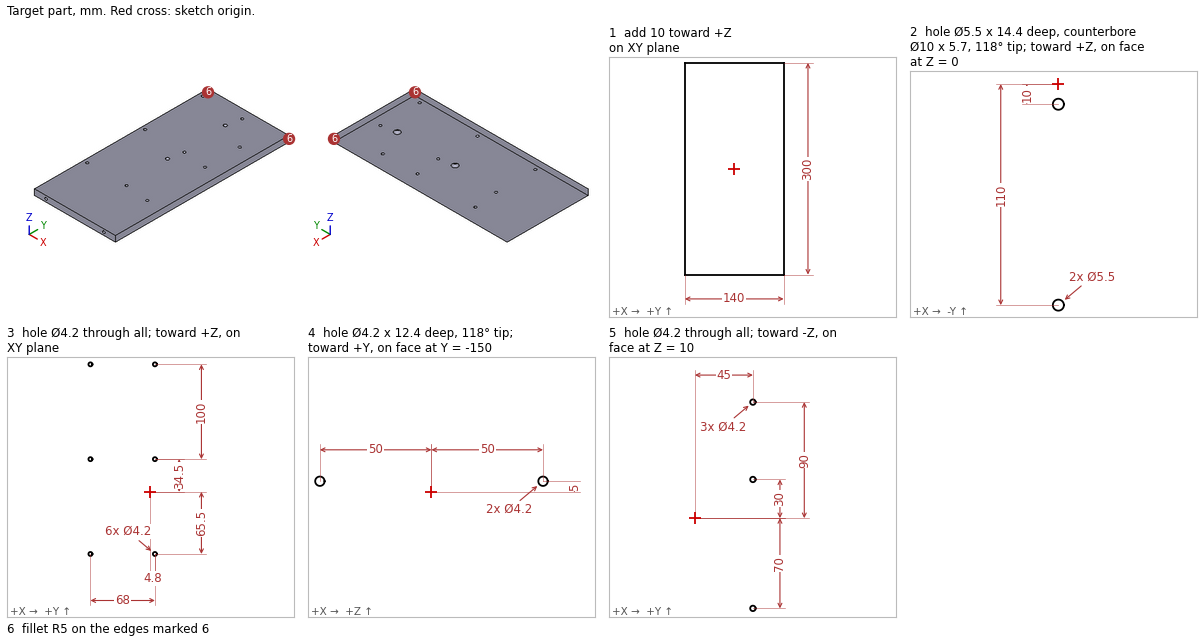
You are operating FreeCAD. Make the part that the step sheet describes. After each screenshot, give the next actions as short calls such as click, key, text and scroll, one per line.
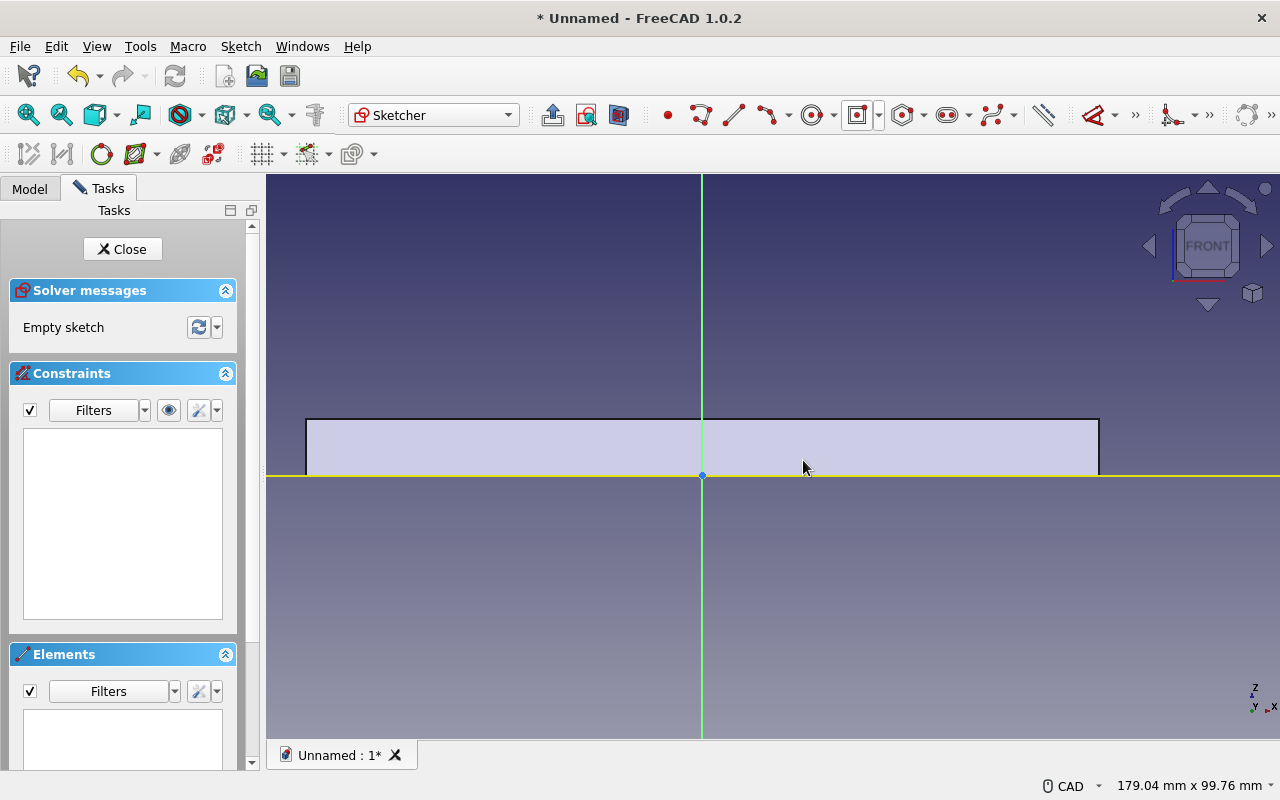
click(812, 116)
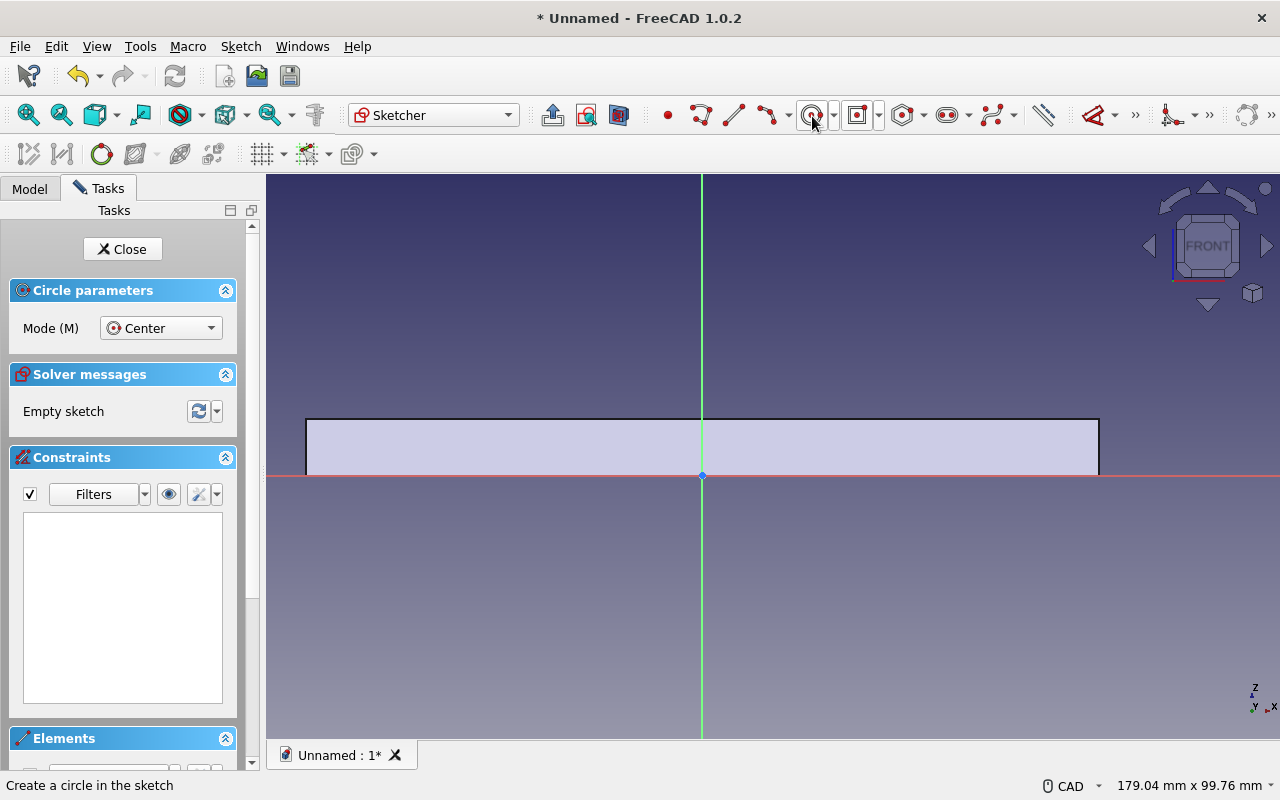
scroll(985, 447, up, 4)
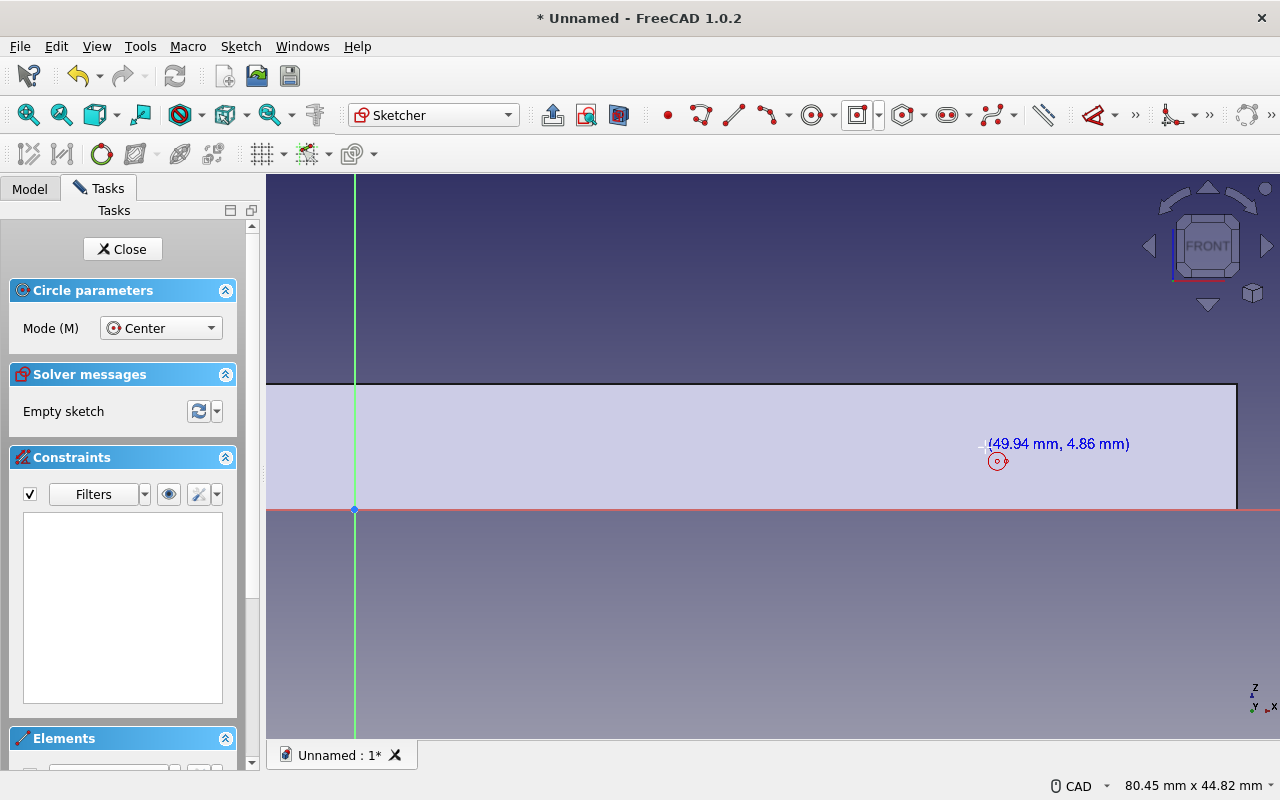
click(985, 447)
click(1004, 428)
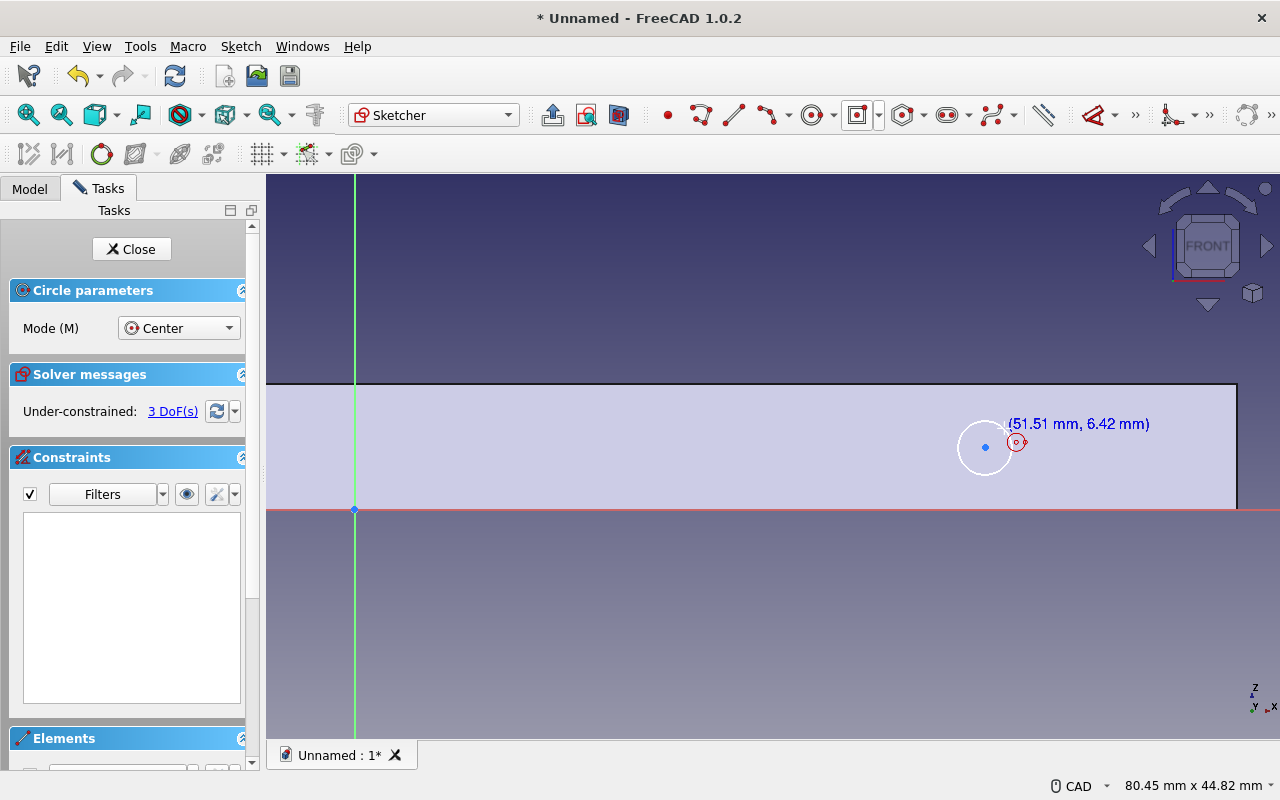
scroll(990, 449, down, 4)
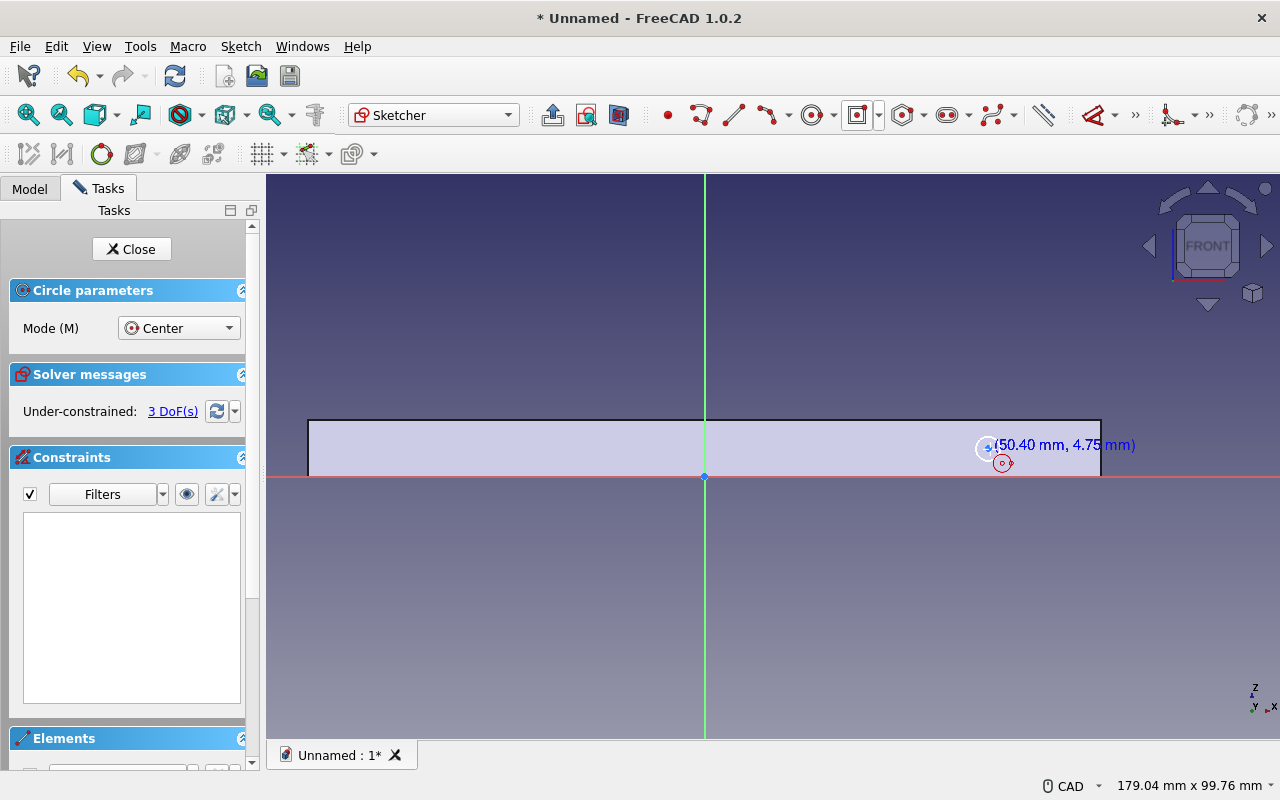
scroll(422, 448, up, 4)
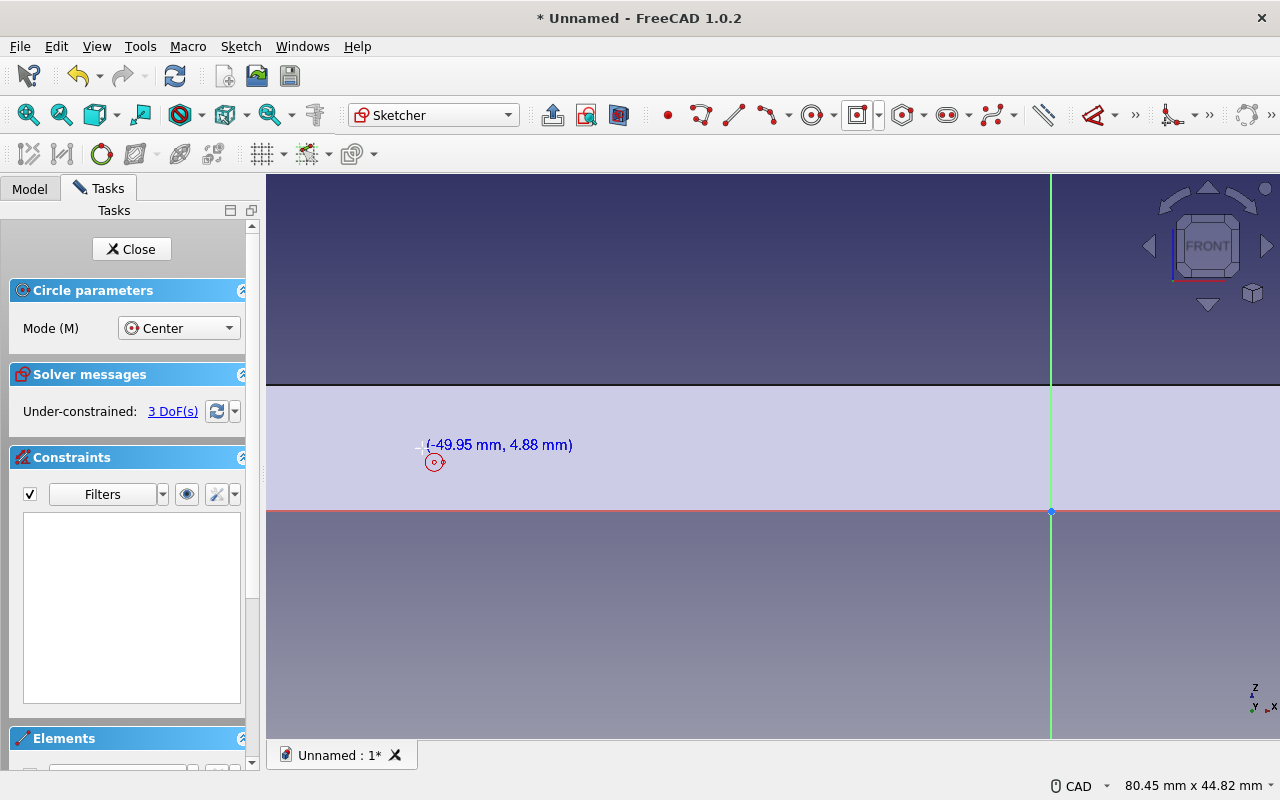
click(421, 448)
click(440, 429)
key(Escape)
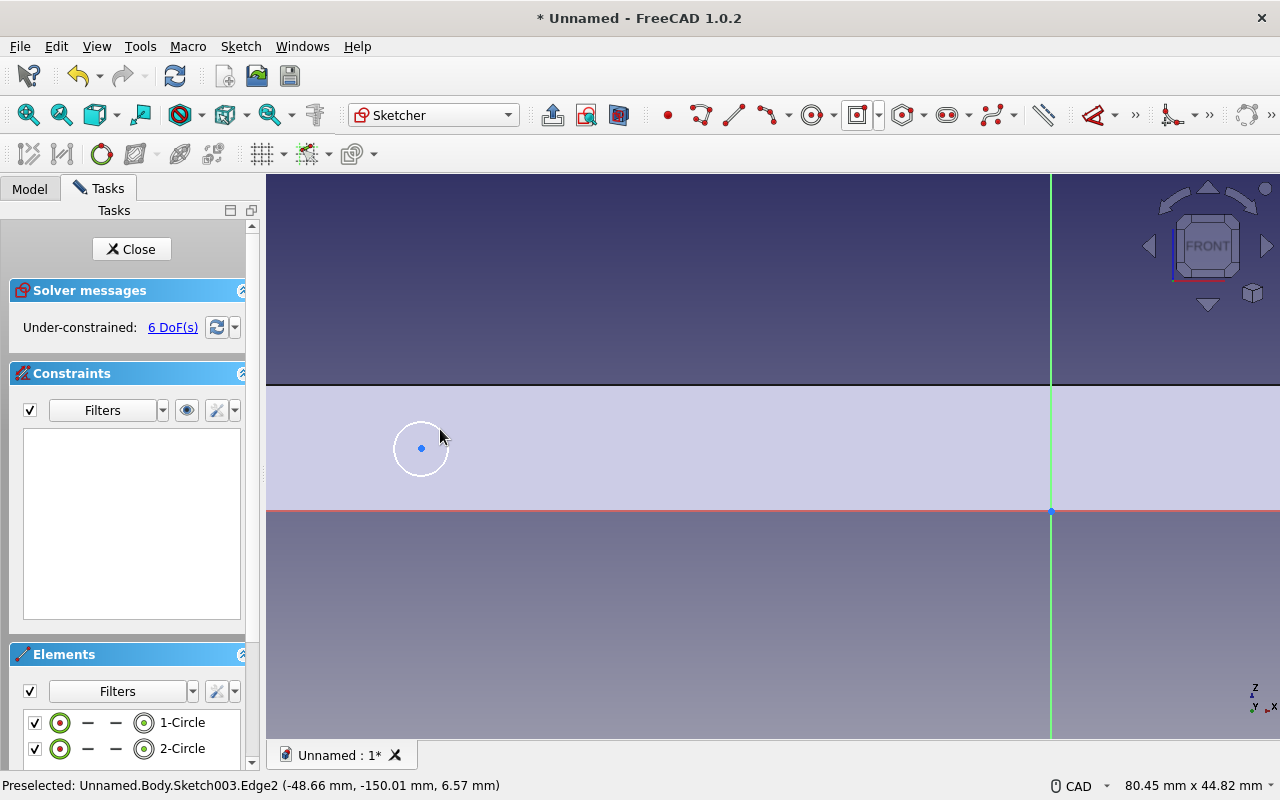
scroll(421, 448, down, 4)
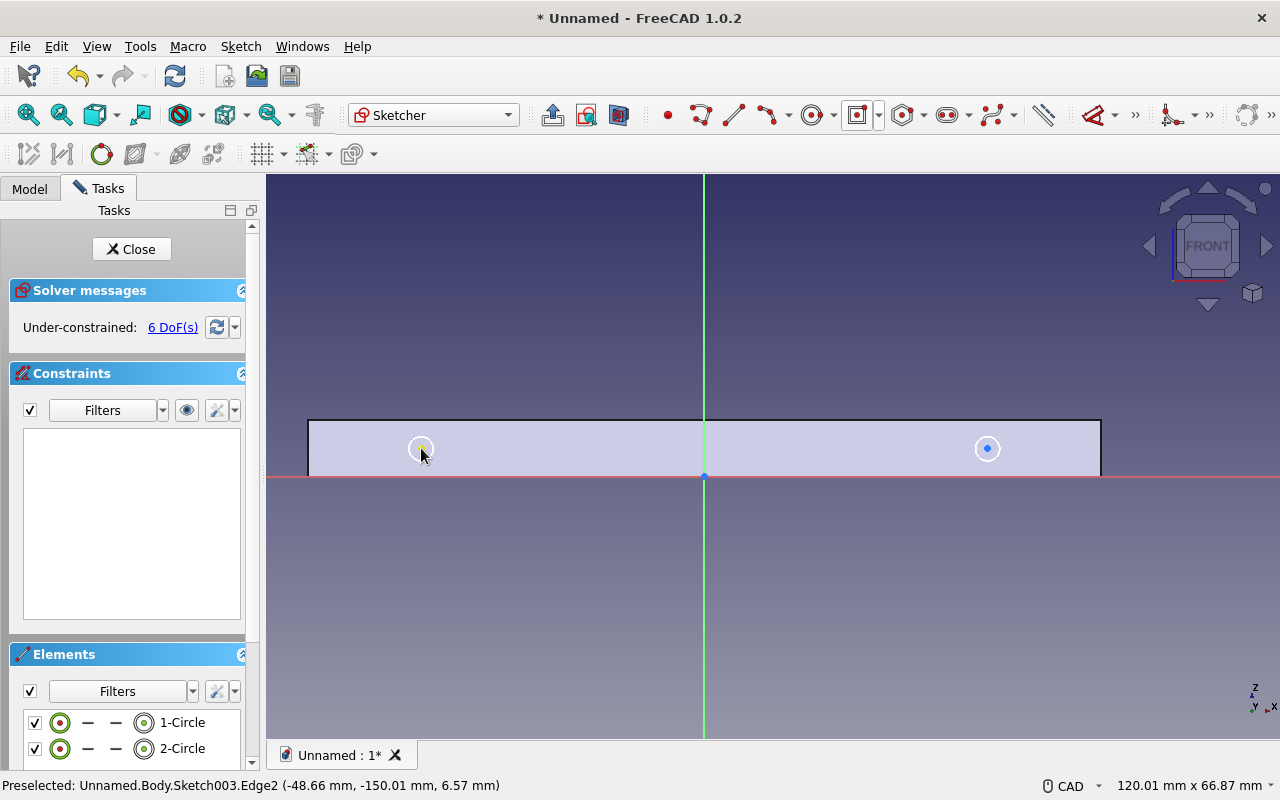
click(996, 440)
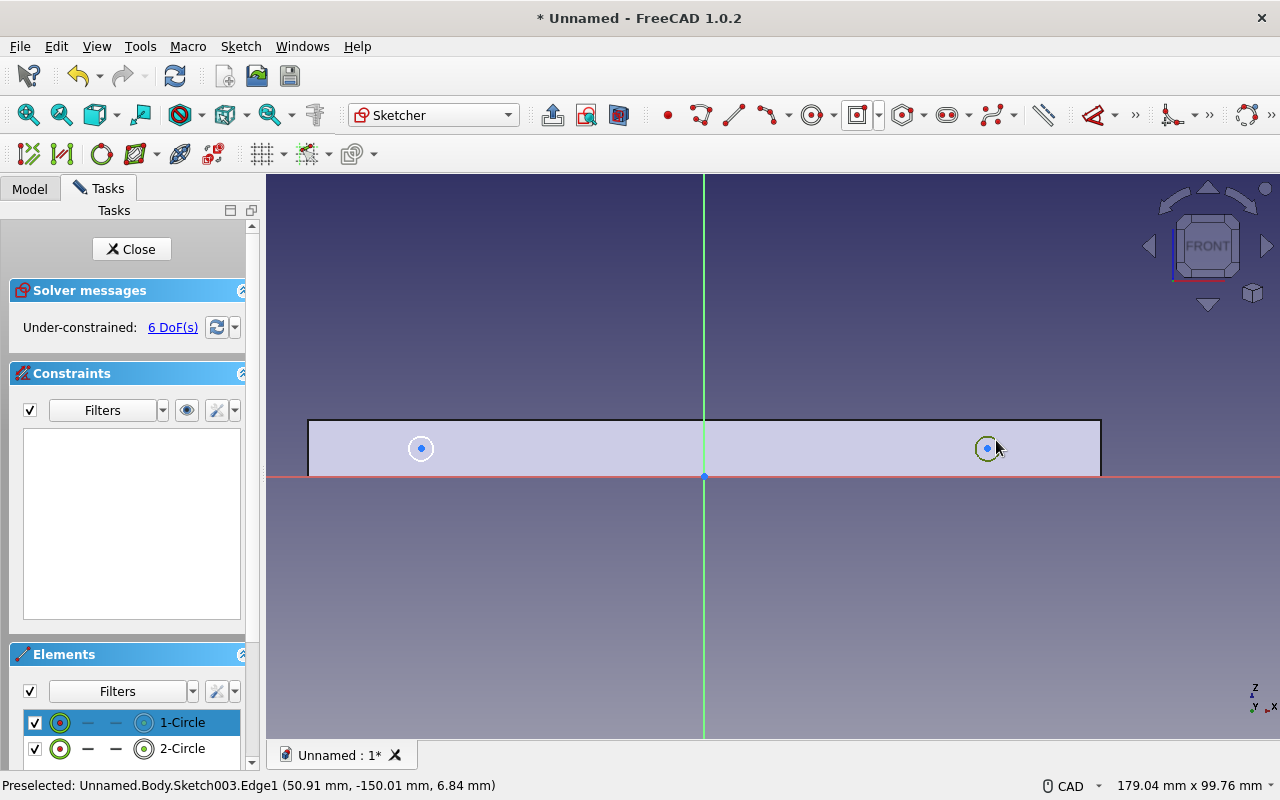
click(430, 440)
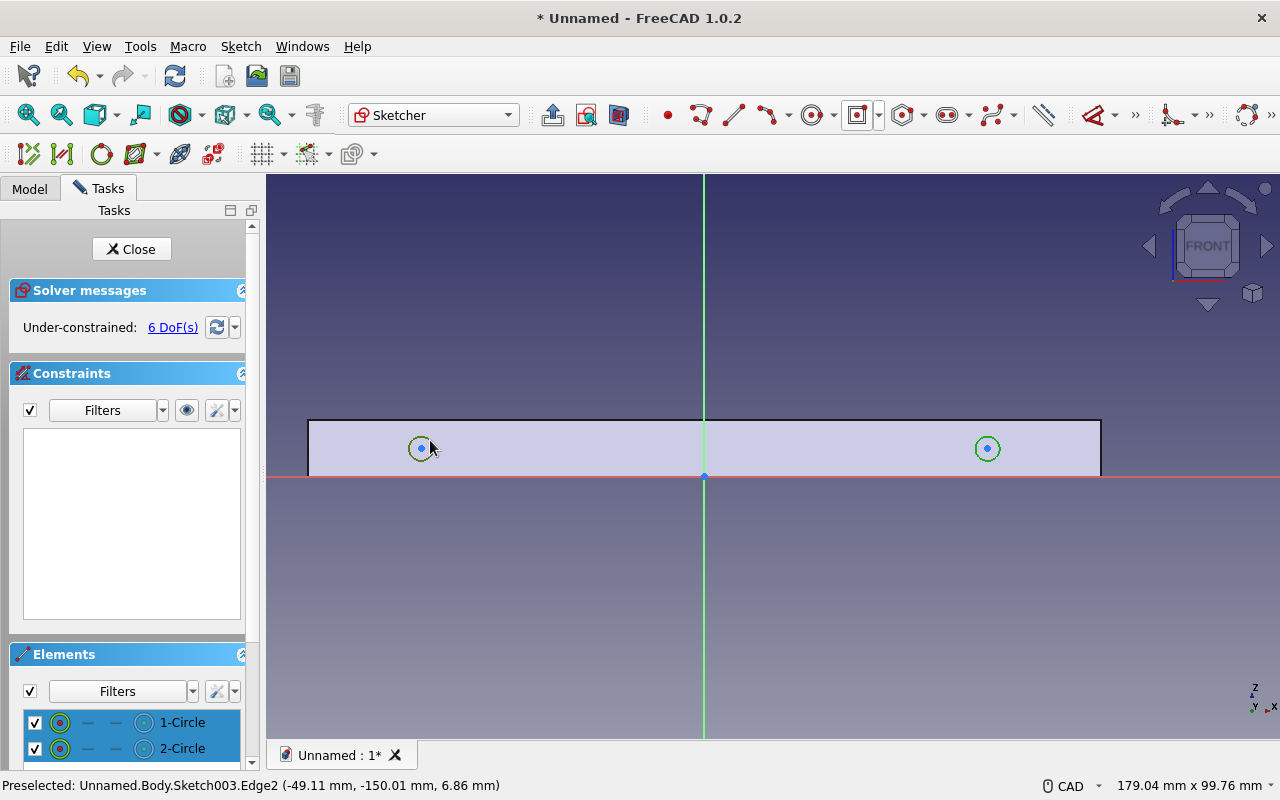
key(e)